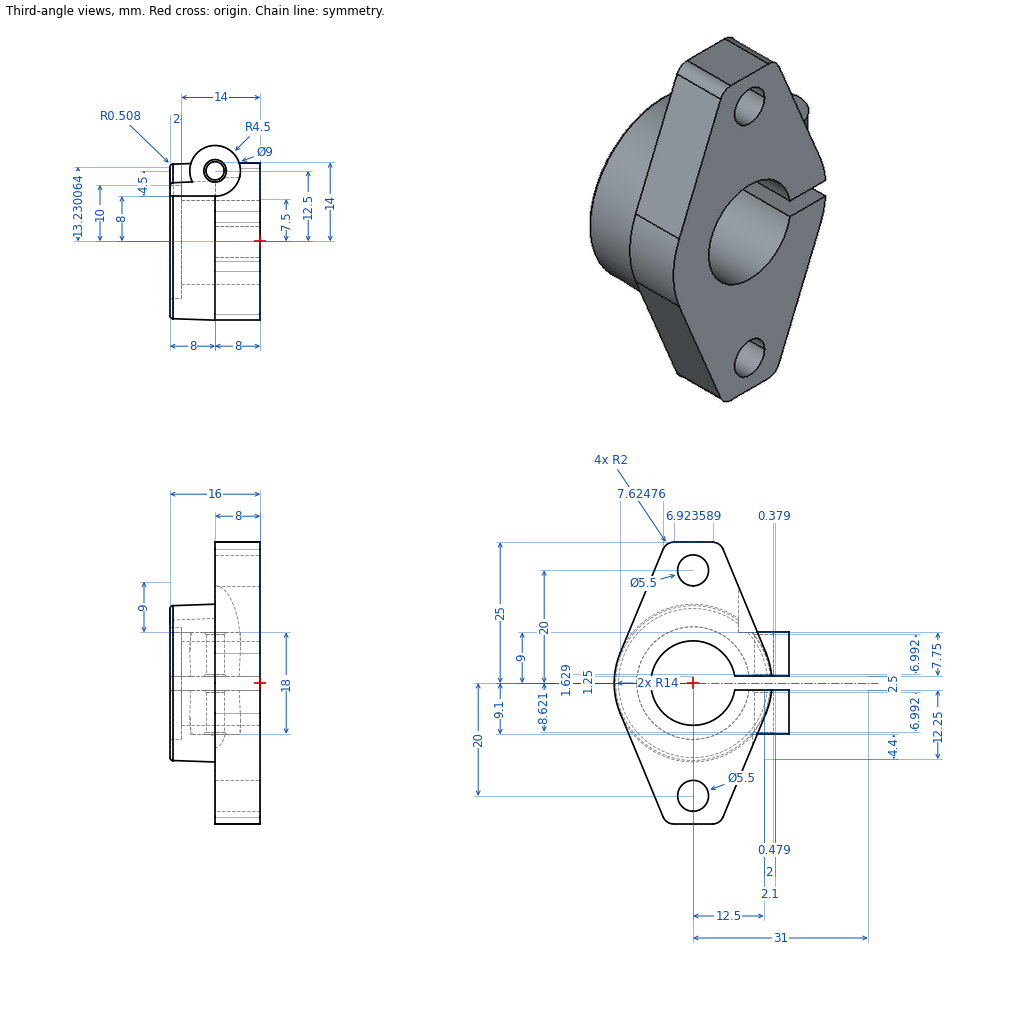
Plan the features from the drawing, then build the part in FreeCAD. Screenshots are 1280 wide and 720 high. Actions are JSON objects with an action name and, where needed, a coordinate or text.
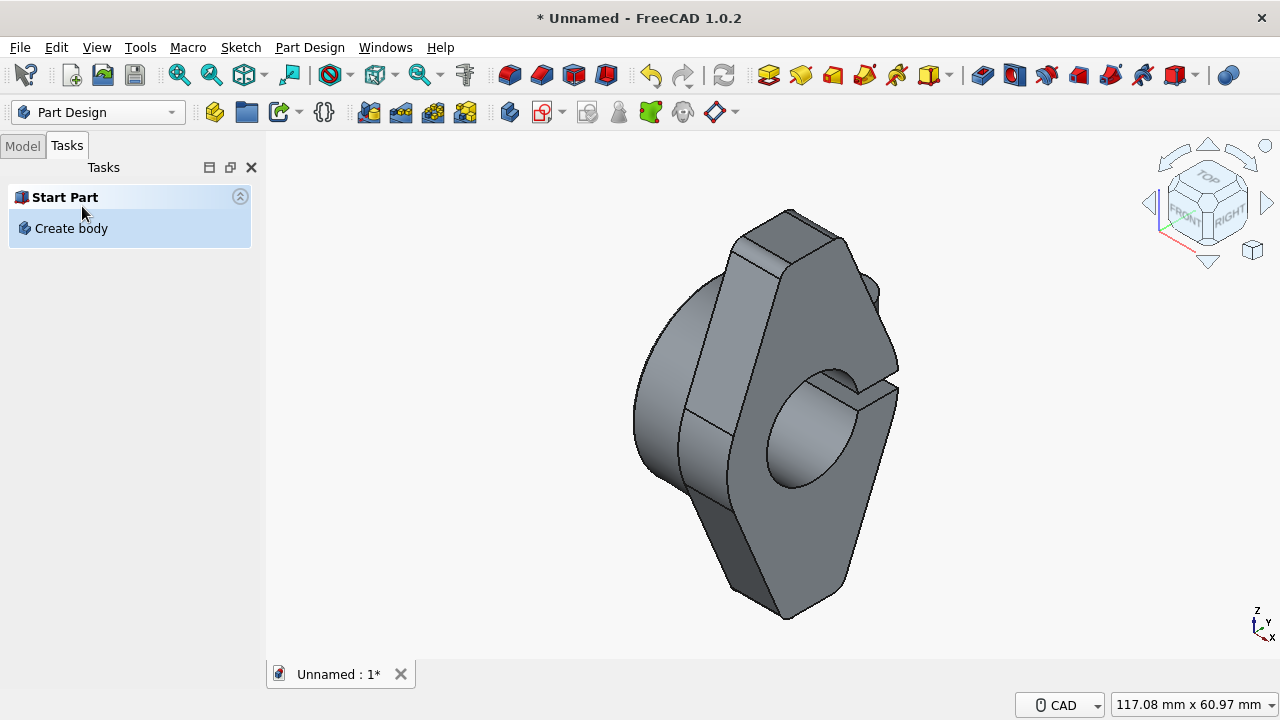
{"action": "key", "text": "6"}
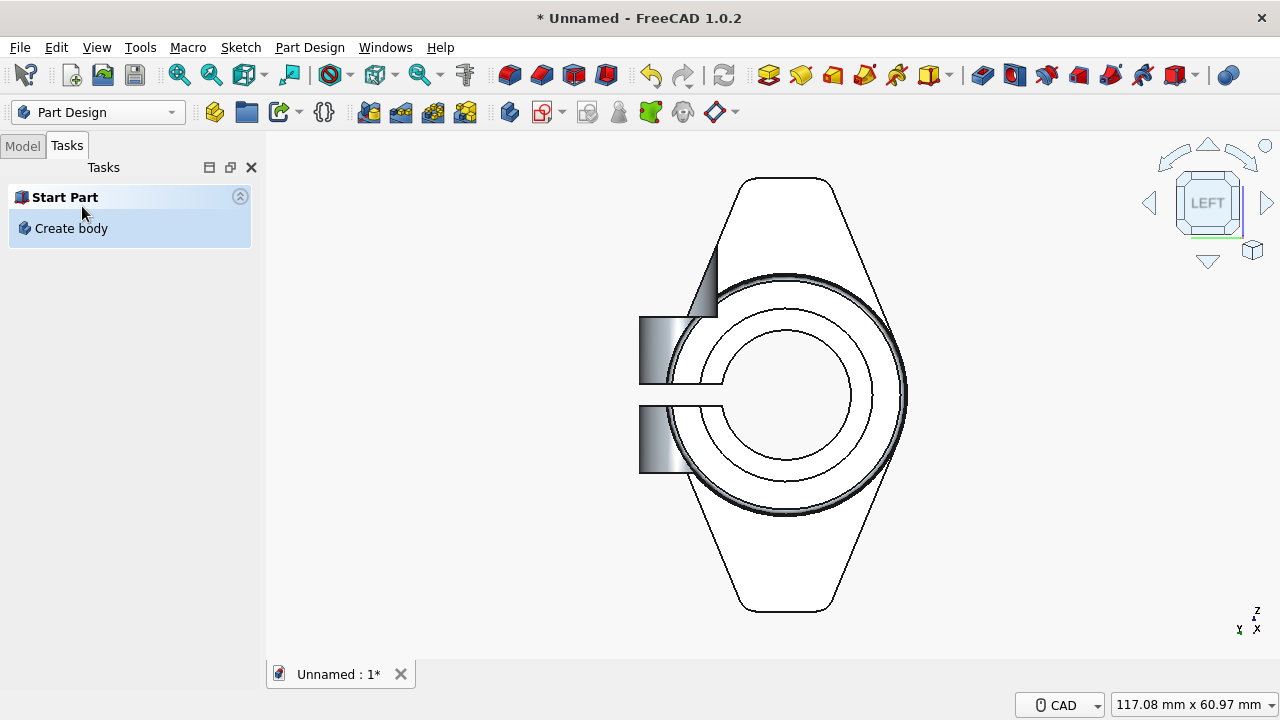
{"action": "left_click", "coordinate": [793, 574]}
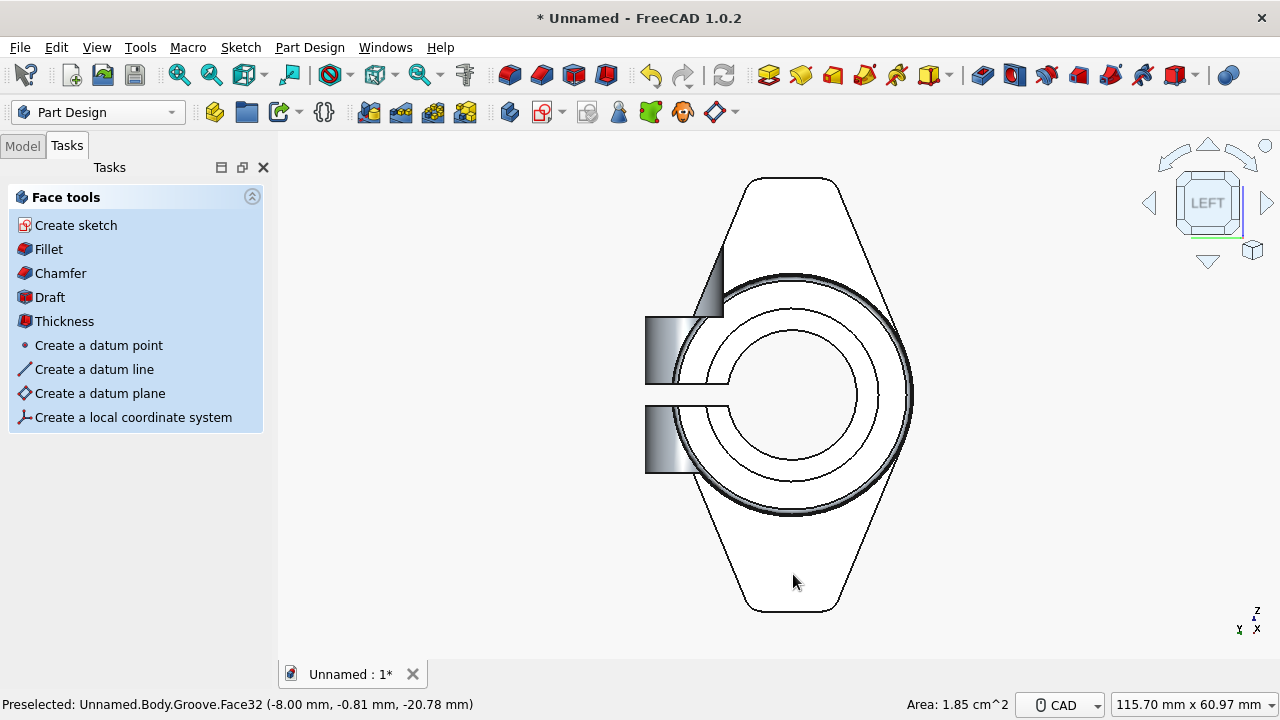
{"action": "left_click", "coordinate": [542, 112]}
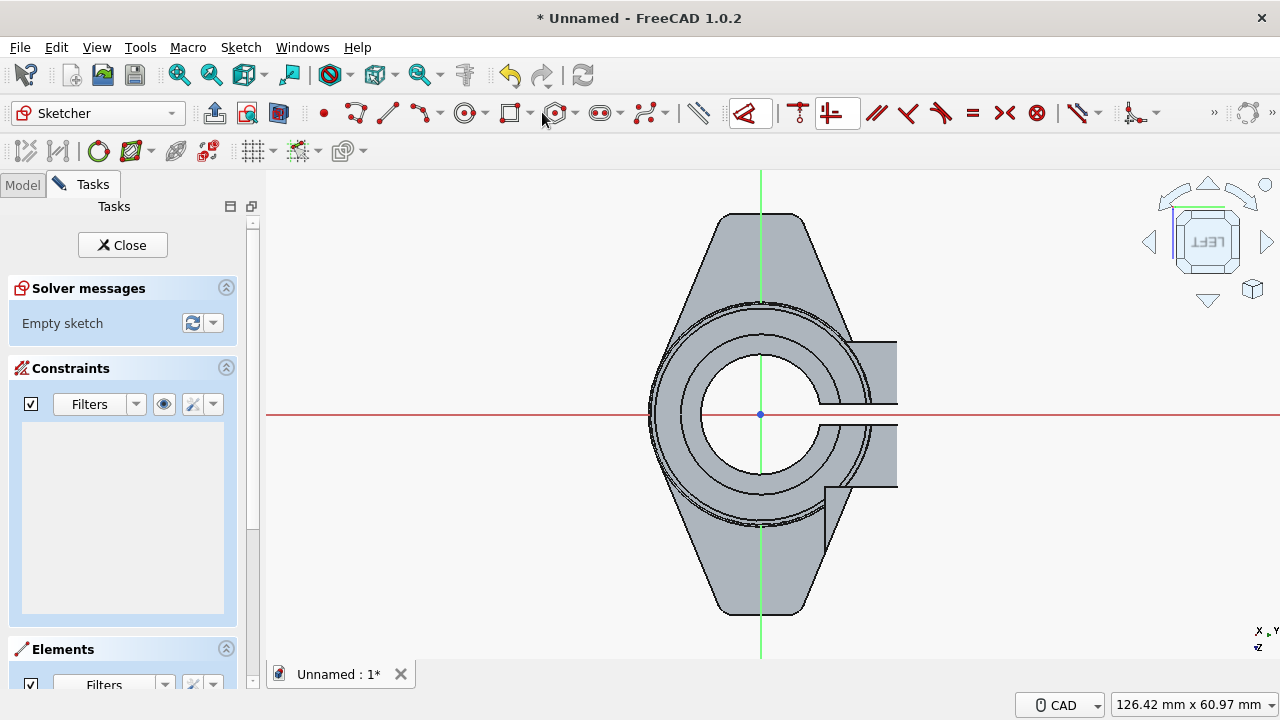
{"action": "left_click", "coordinate": [280, 114]}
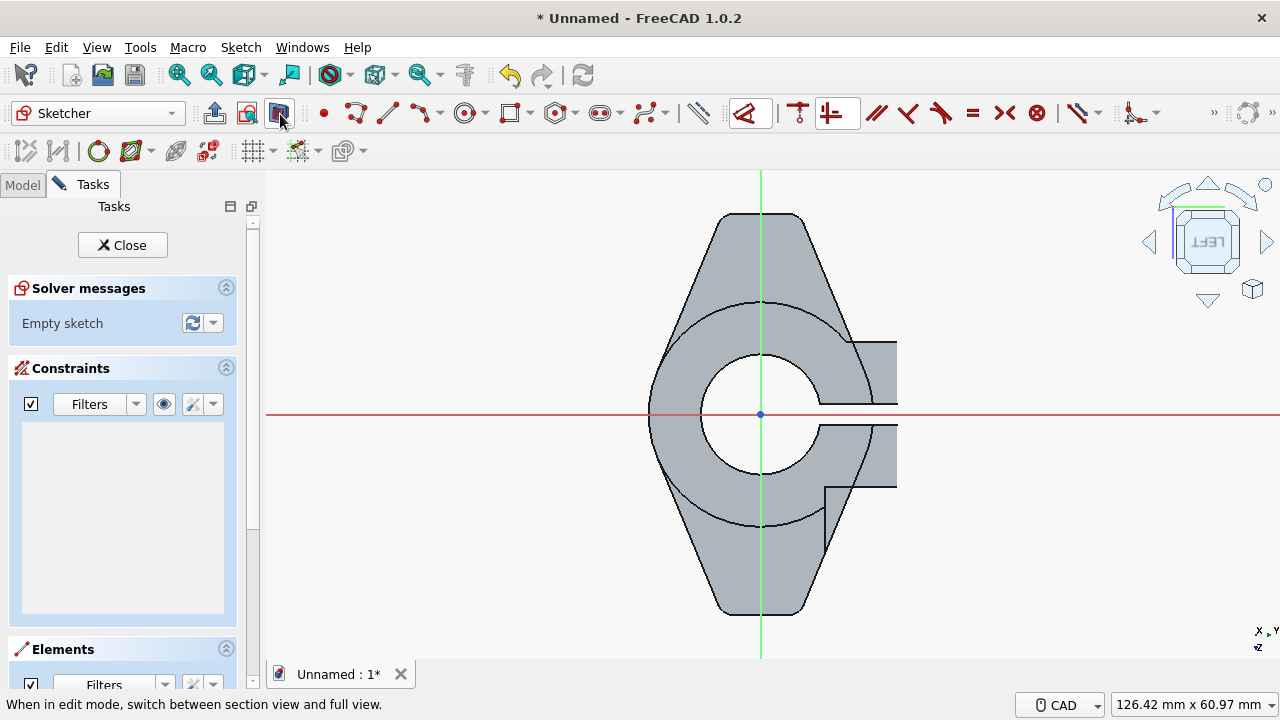
{"action": "scroll", "coordinate": [913, 343], "scroll_direction": "up", "scroll_amount": 4}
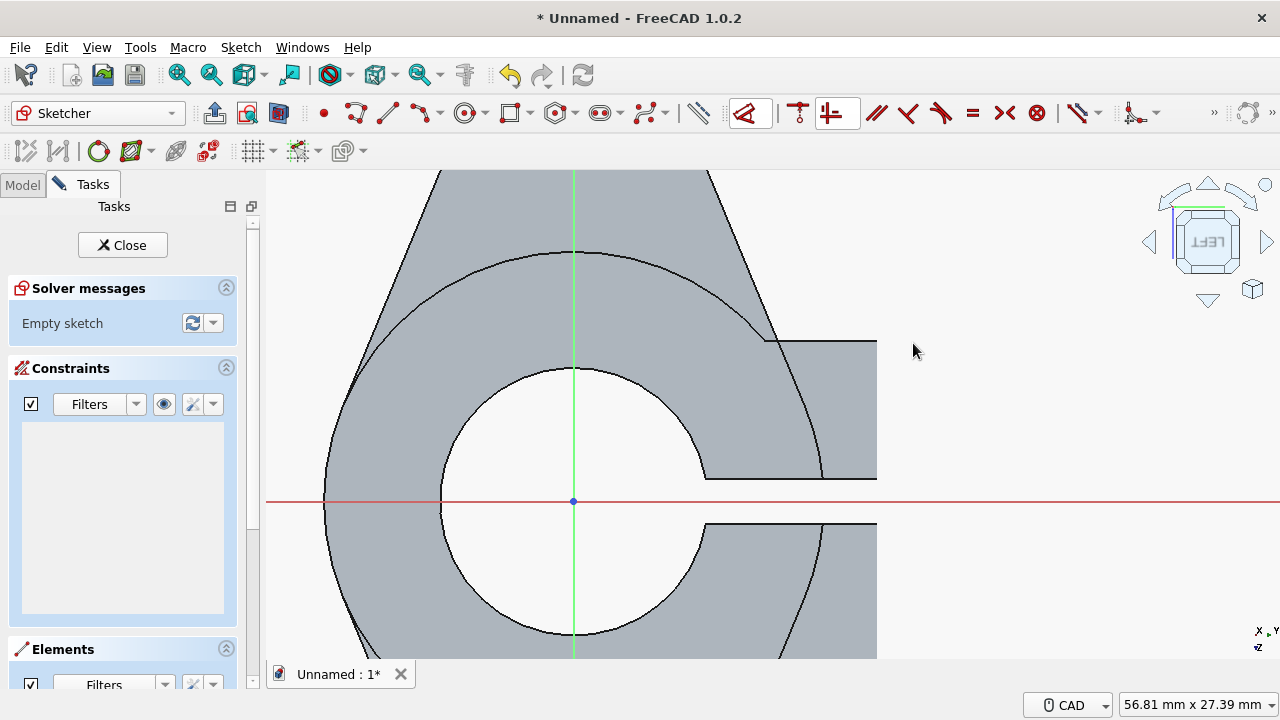
{"action": "left_click", "coordinate": [356, 114]}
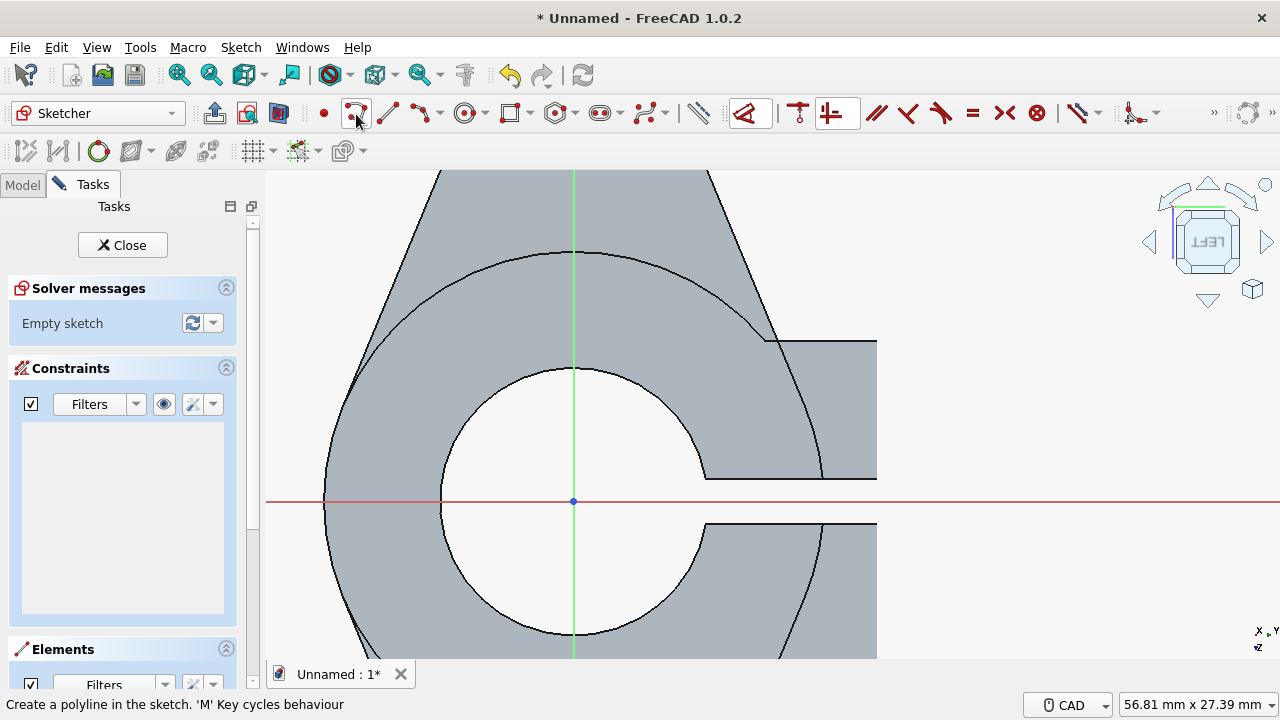
{"action": "left_click", "coordinate": [797, 479]}
{"action": "left_click", "coordinate": [797, 261]}
{"action": "left_click", "coordinate": [834, 261]}
{"action": "left_click", "coordinate": [834, 339]}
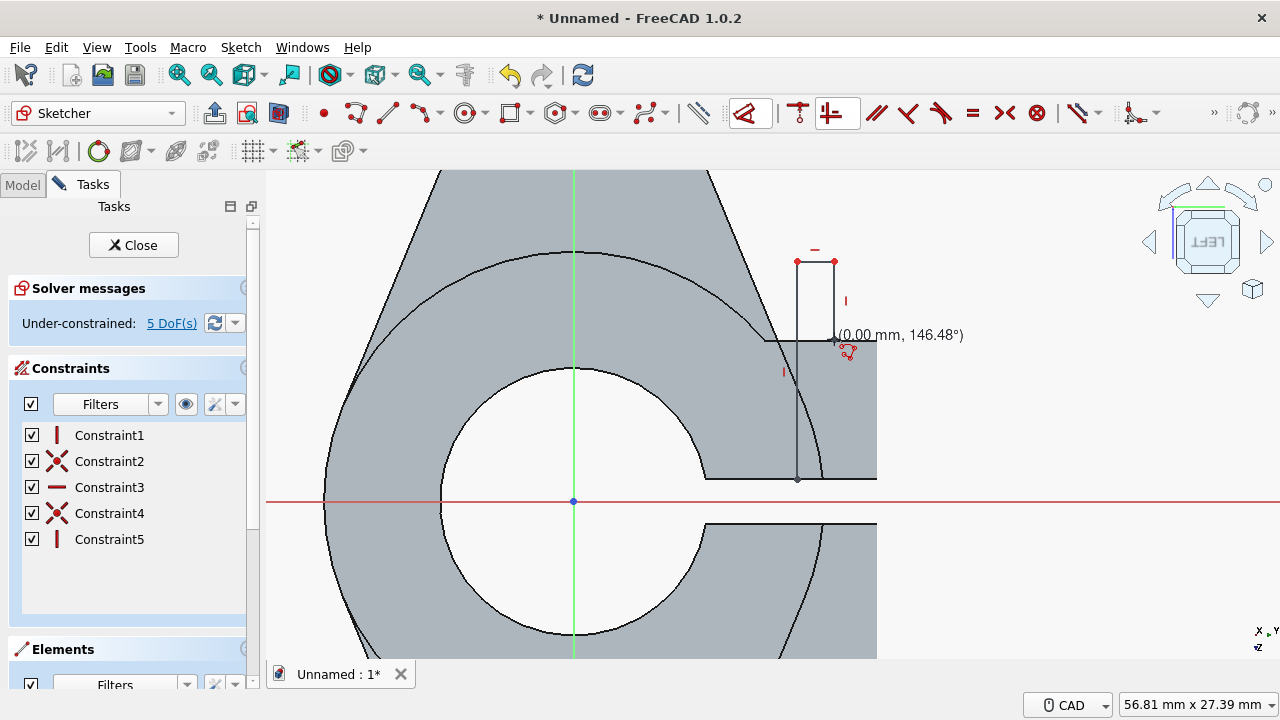
{"action": "scroll", "coordinate": [826, 348], "scroll_direction": "up", "scroll_amount": 2}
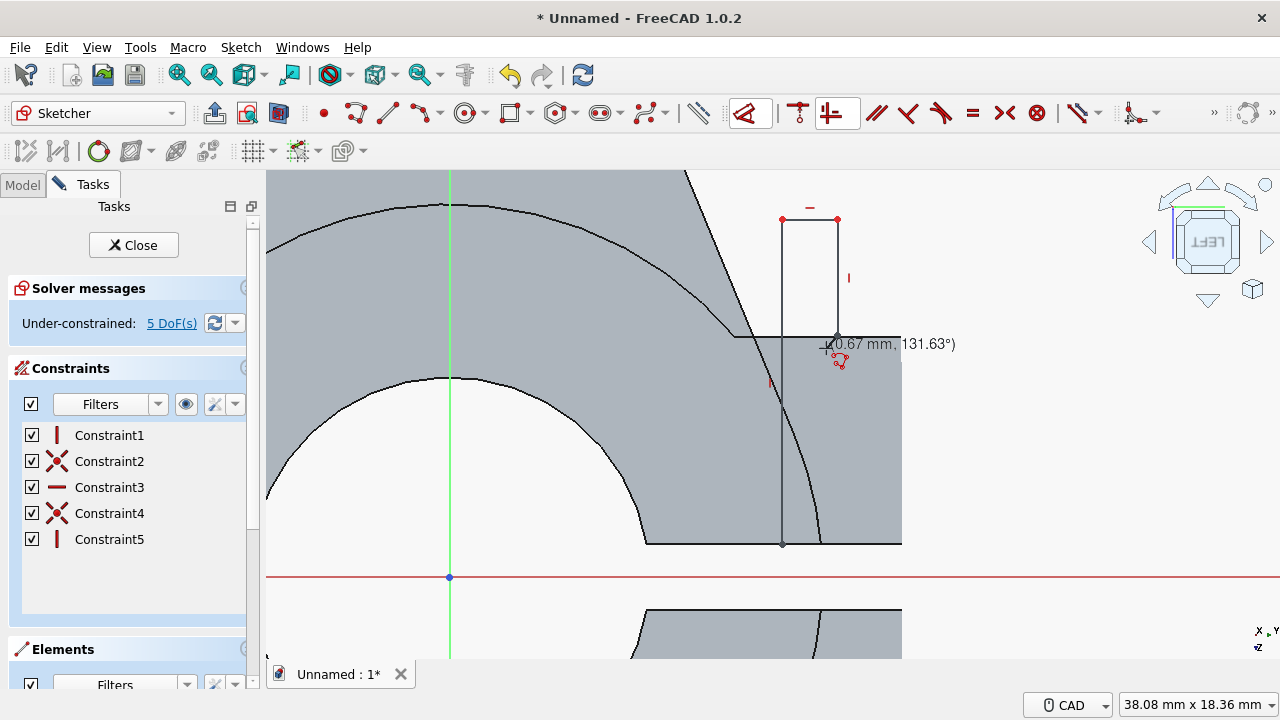
{"action": "left_click", "coordinate": [826, 348]}
{"action": "left_click", "coordinate": [826, 534]}
{"action": "left_click", "coordinate": [836, 544]}
{"action": "left_click", "coordinate": [782, 545]}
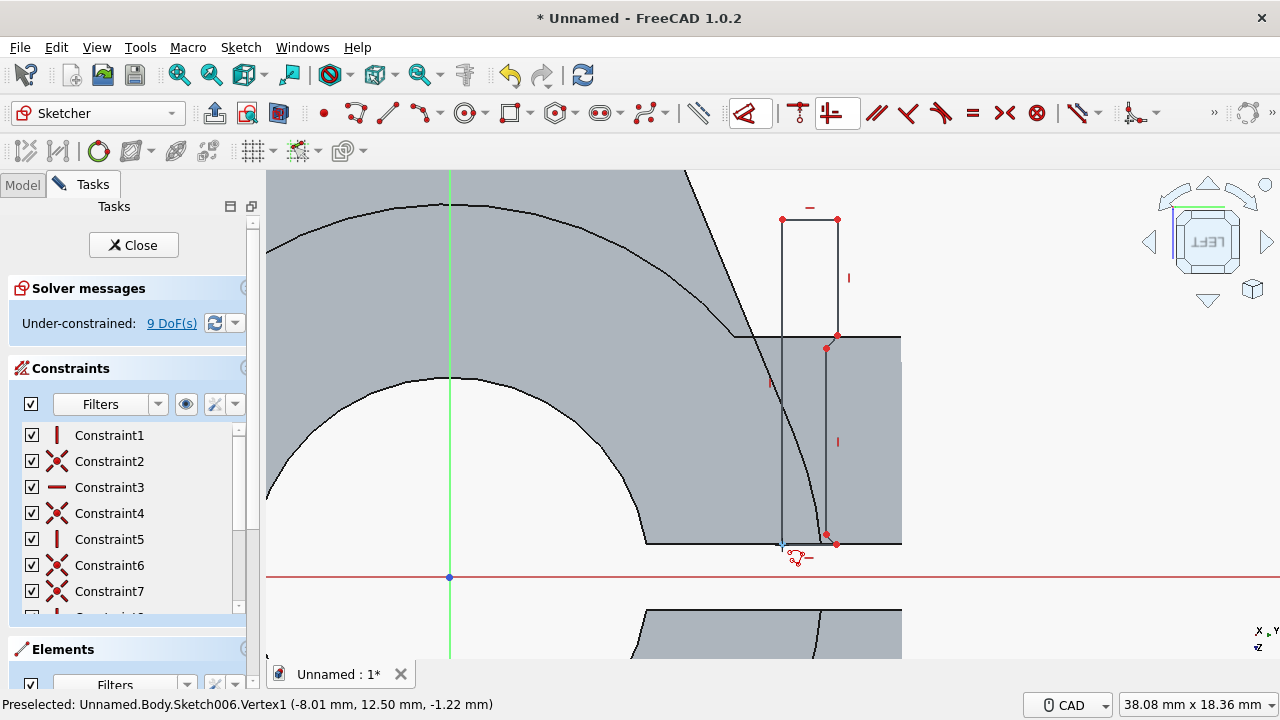
{"action": "left_click", "coordinate": [388, 114]}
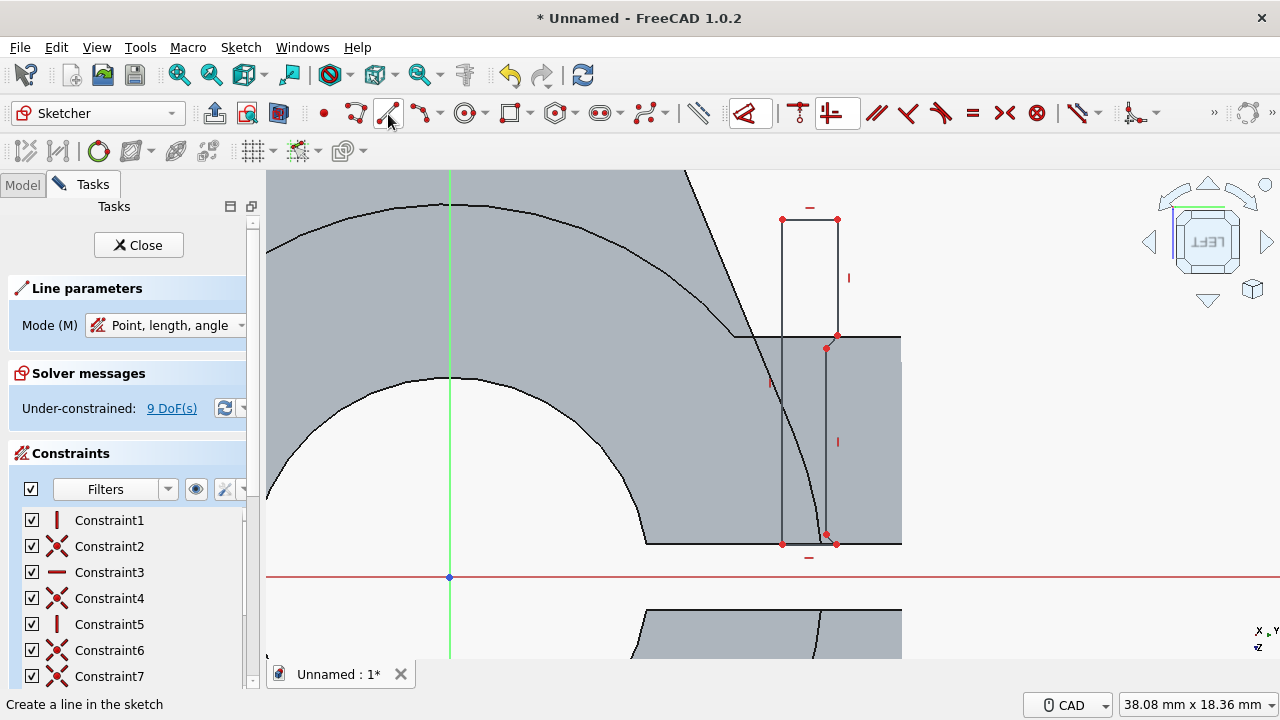
{"action": "scroll", "coordinate": [782, 576], "scroll_direction": "up", "scroll_amount": 16}